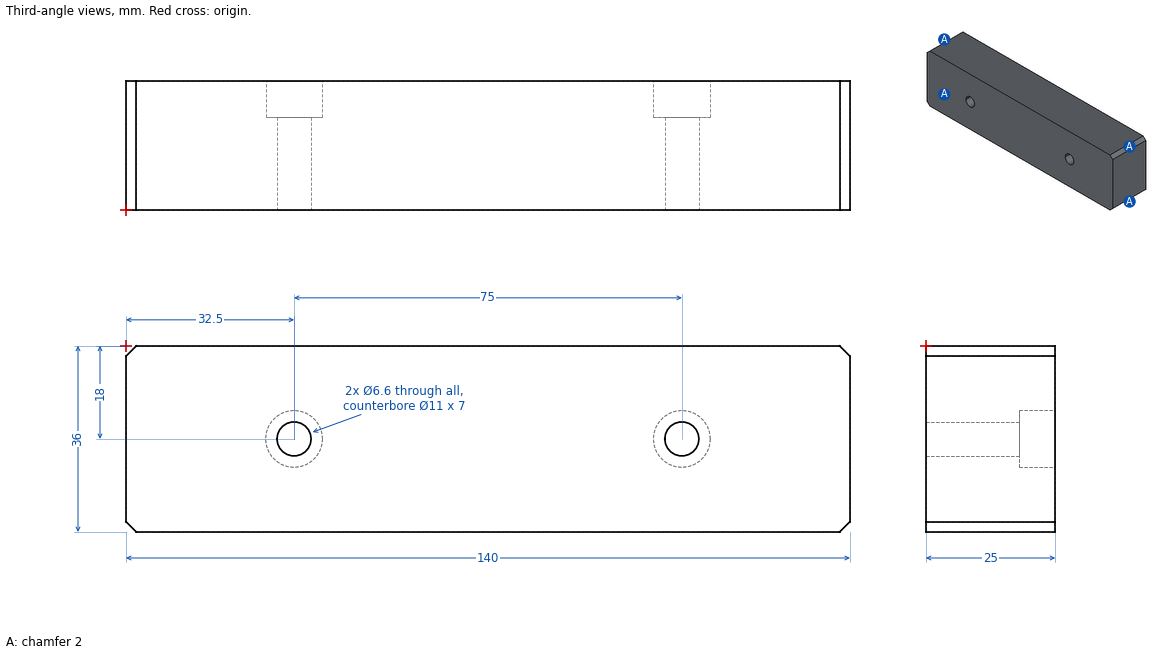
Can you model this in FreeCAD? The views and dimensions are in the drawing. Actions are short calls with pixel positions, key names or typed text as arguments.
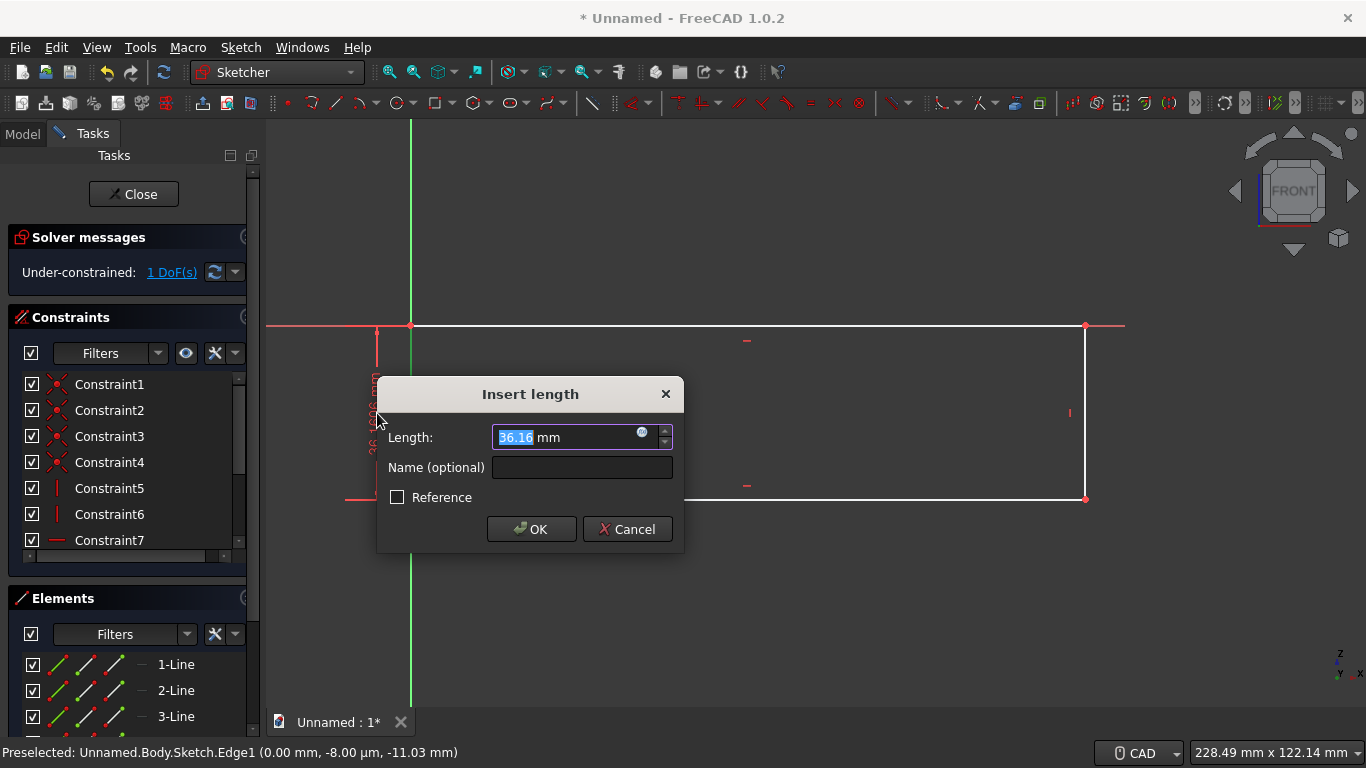
text(36)
key(Return)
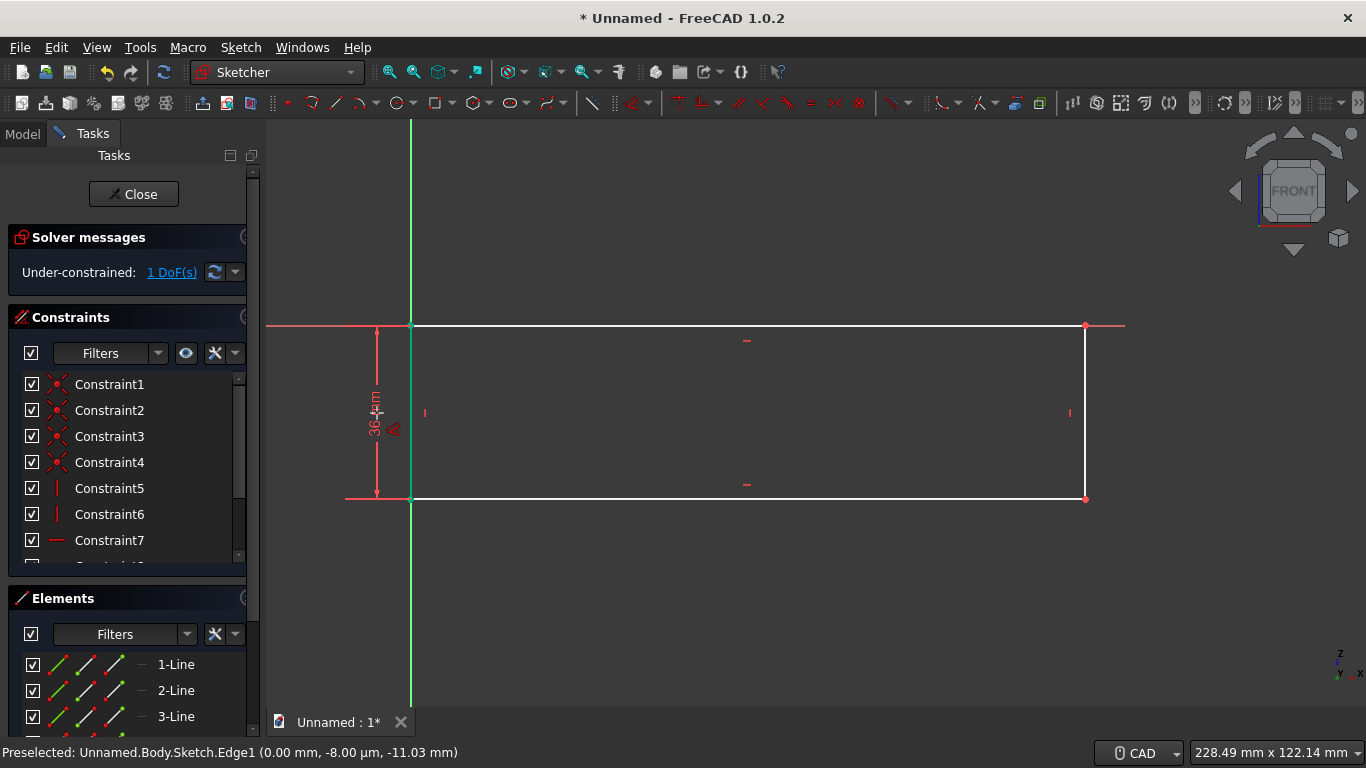
click(613, 499)
click(748, 533)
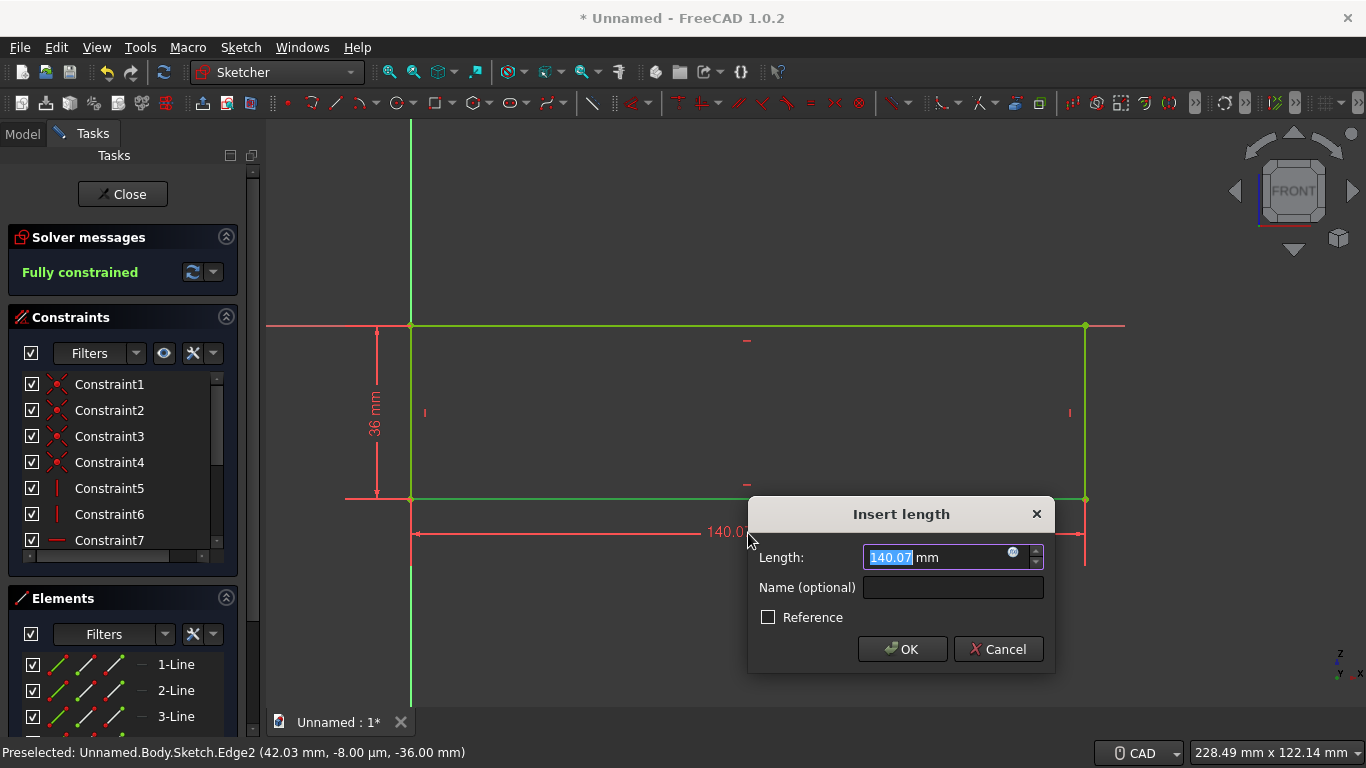
text(140)
key(Return)
key(Escape)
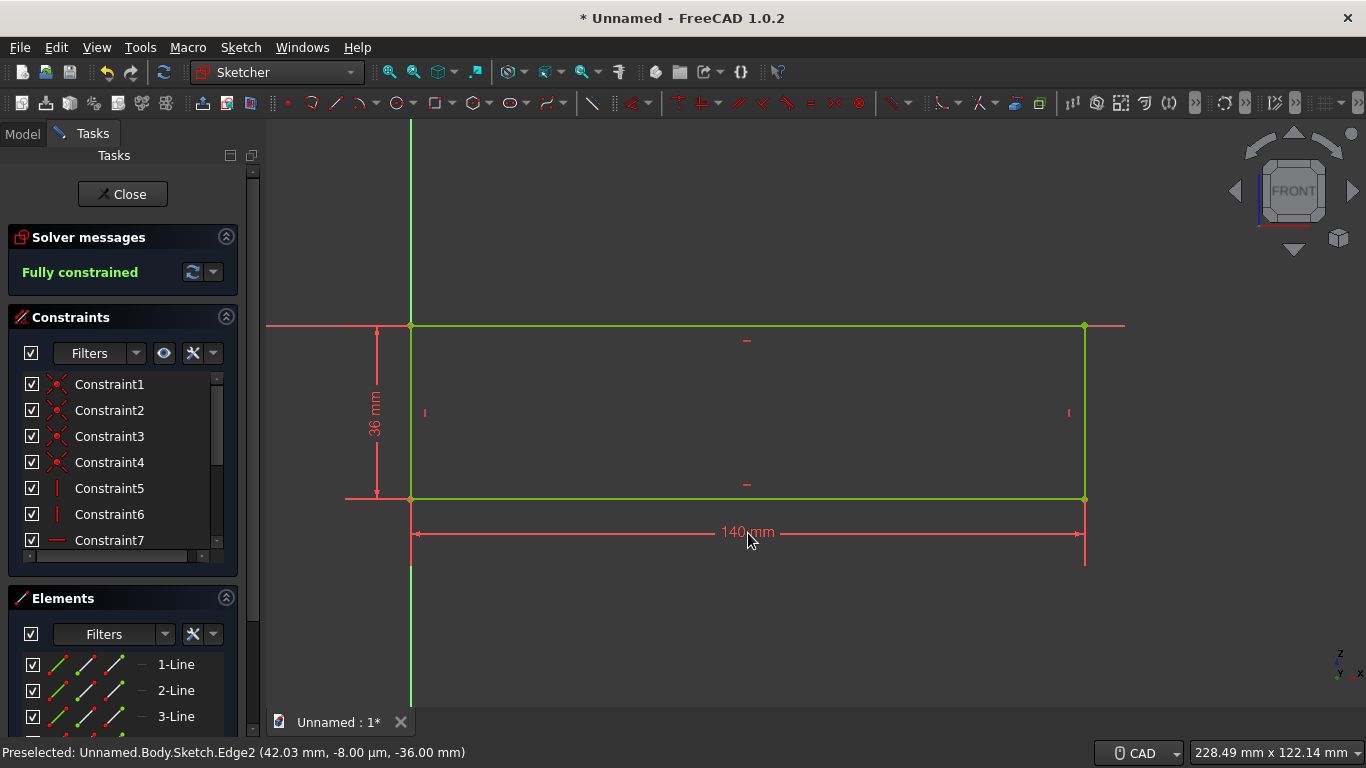
click(123, 194)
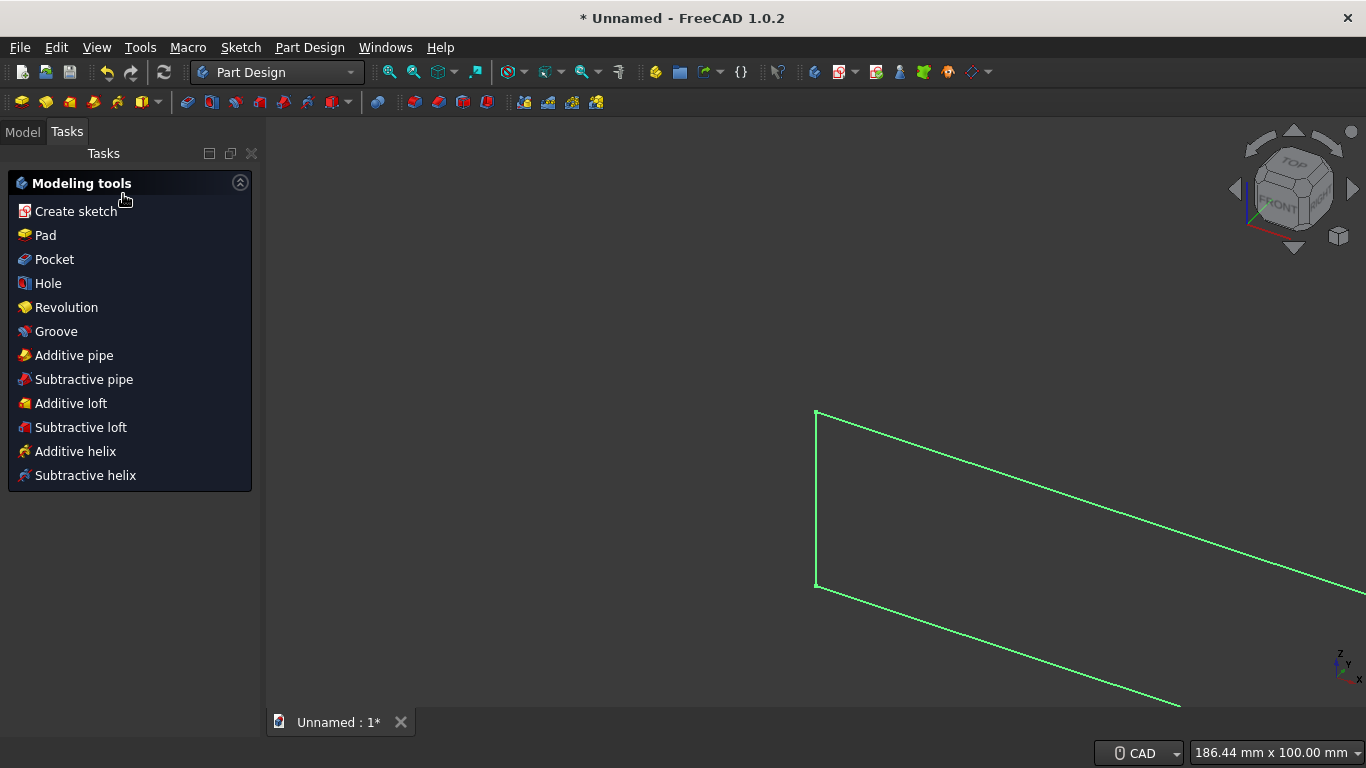
click(22, 102)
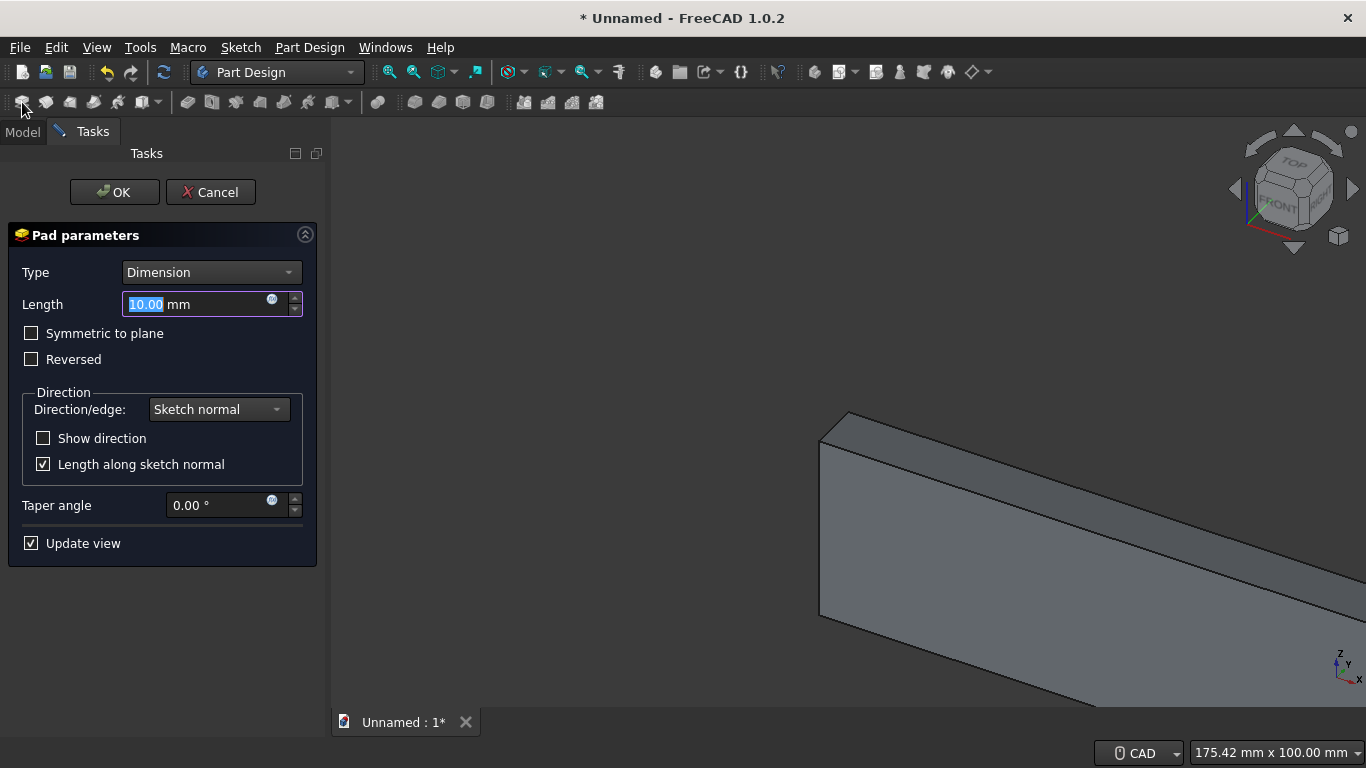
text(25)
key(Tab)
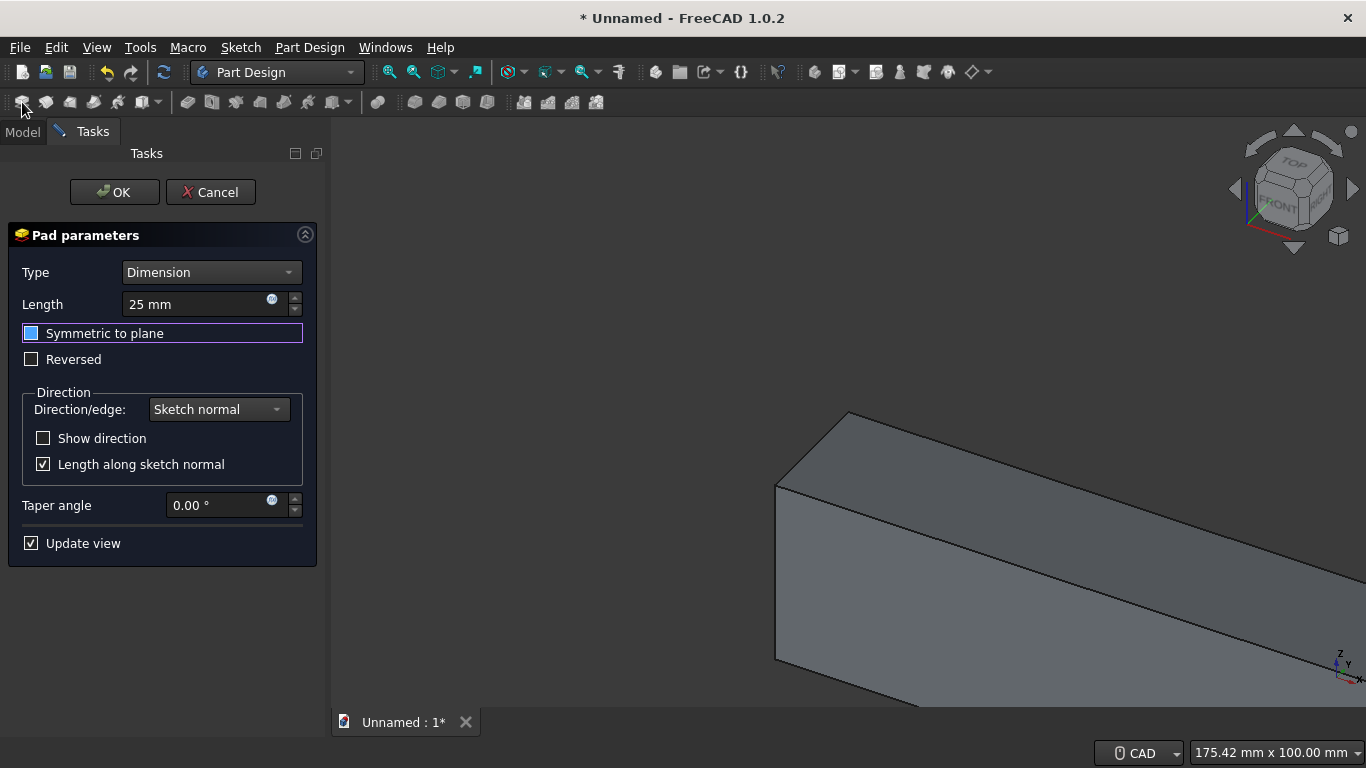
click(30, 359)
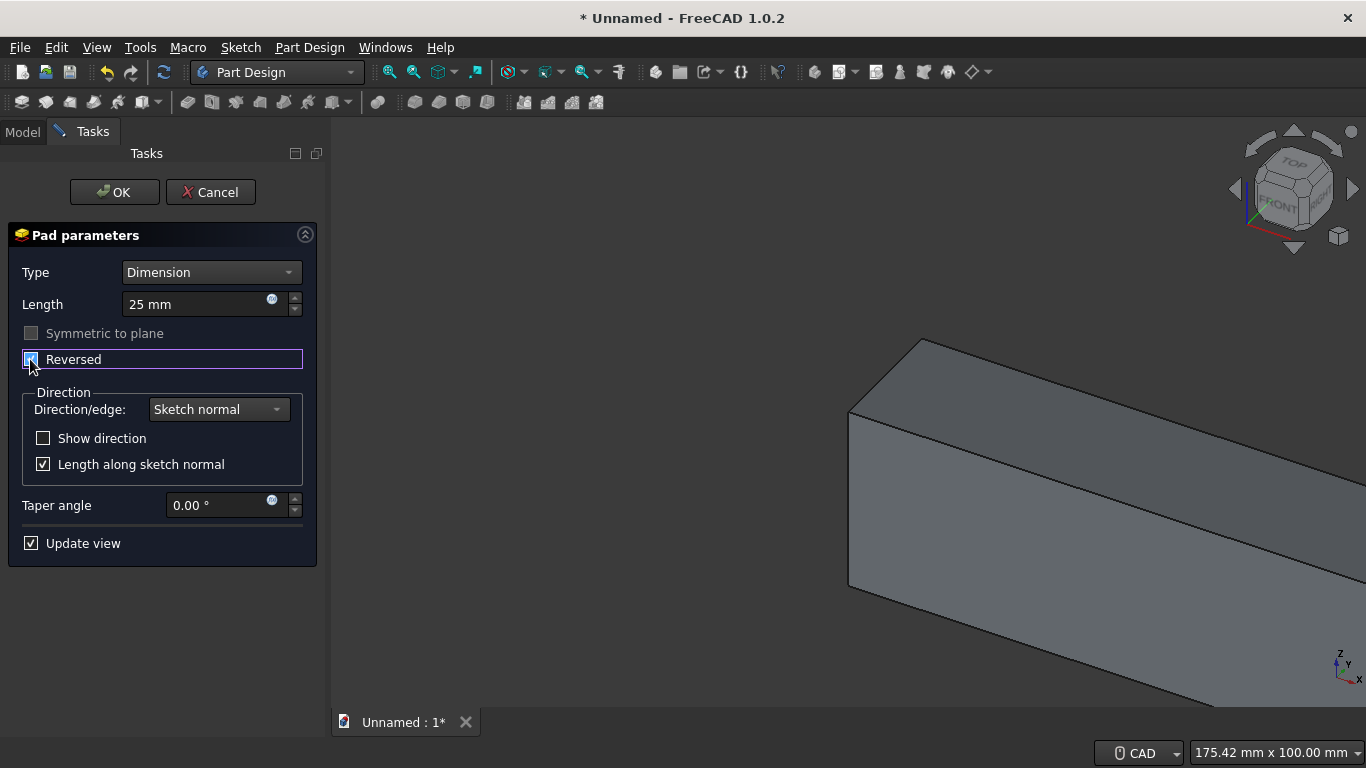
click(115, 192)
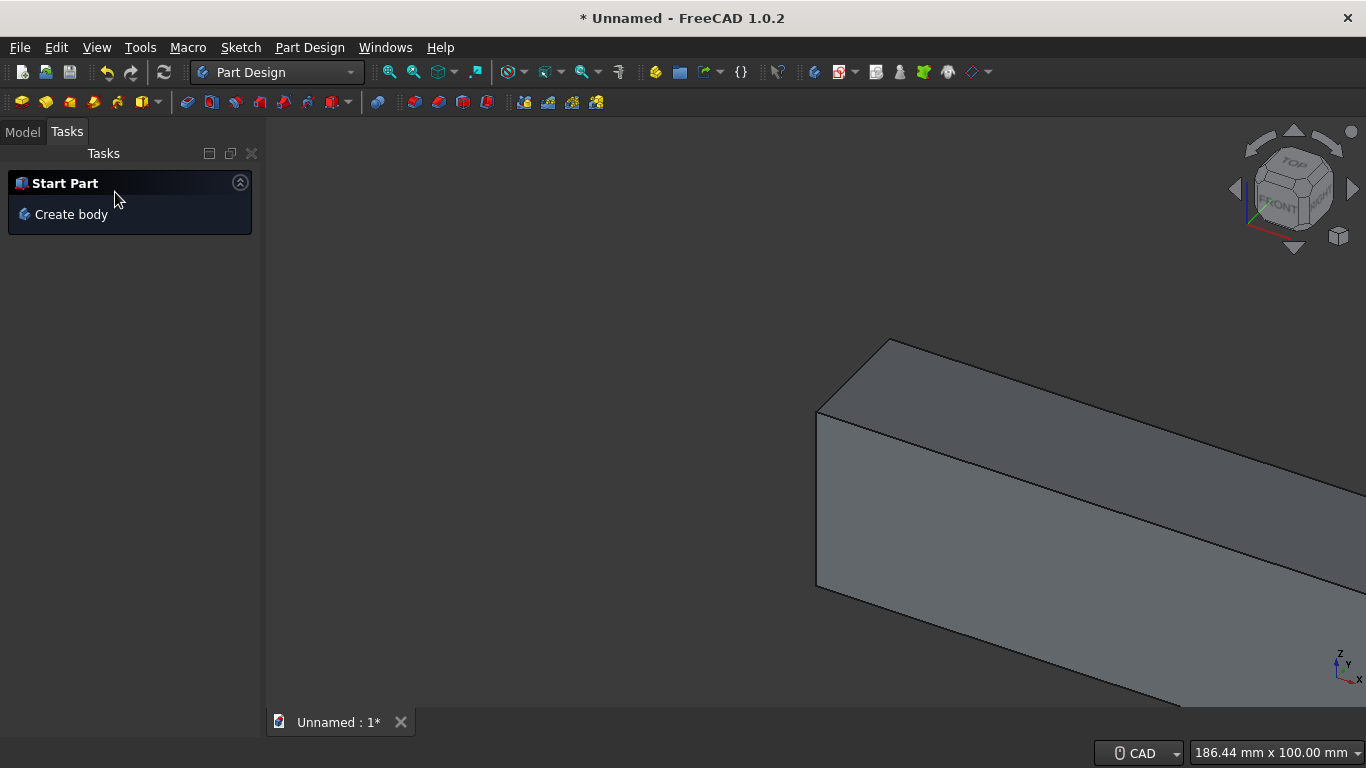
click(390, 72)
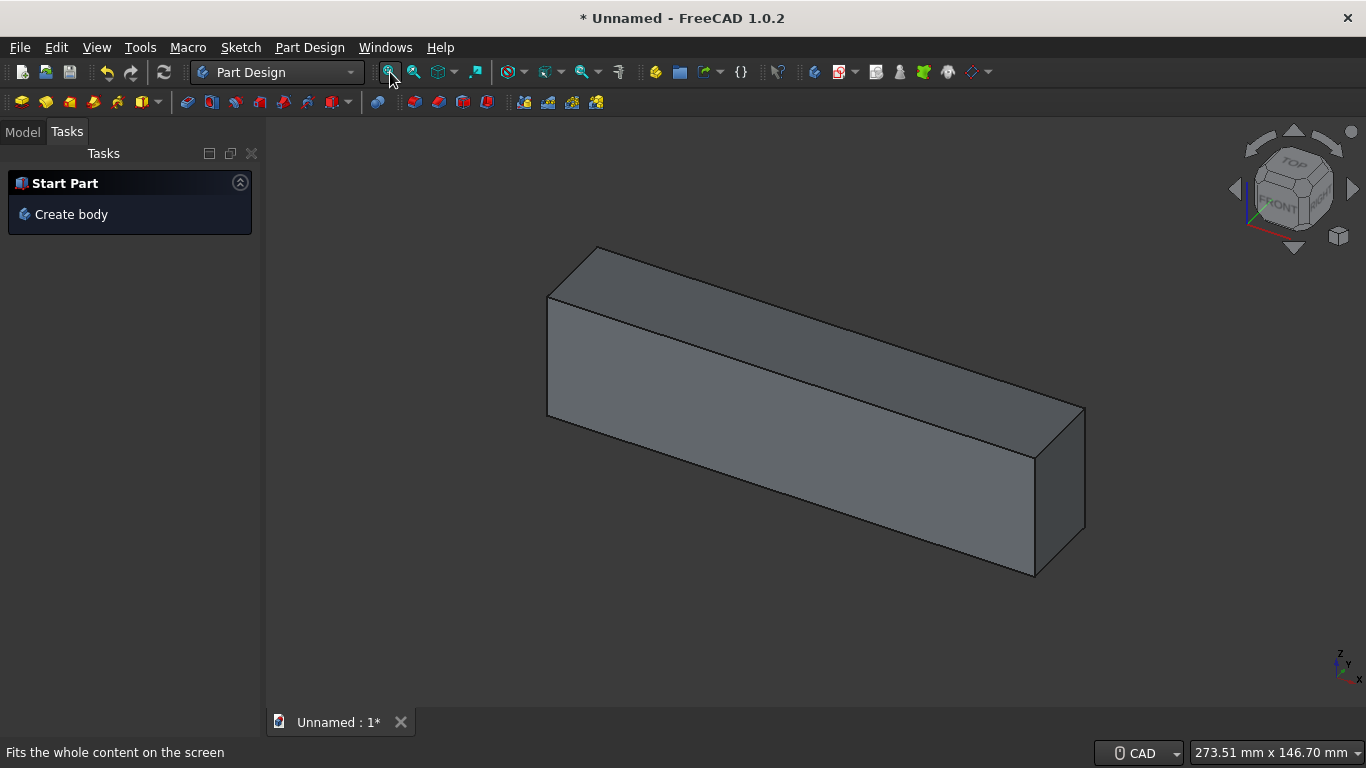
key(4)